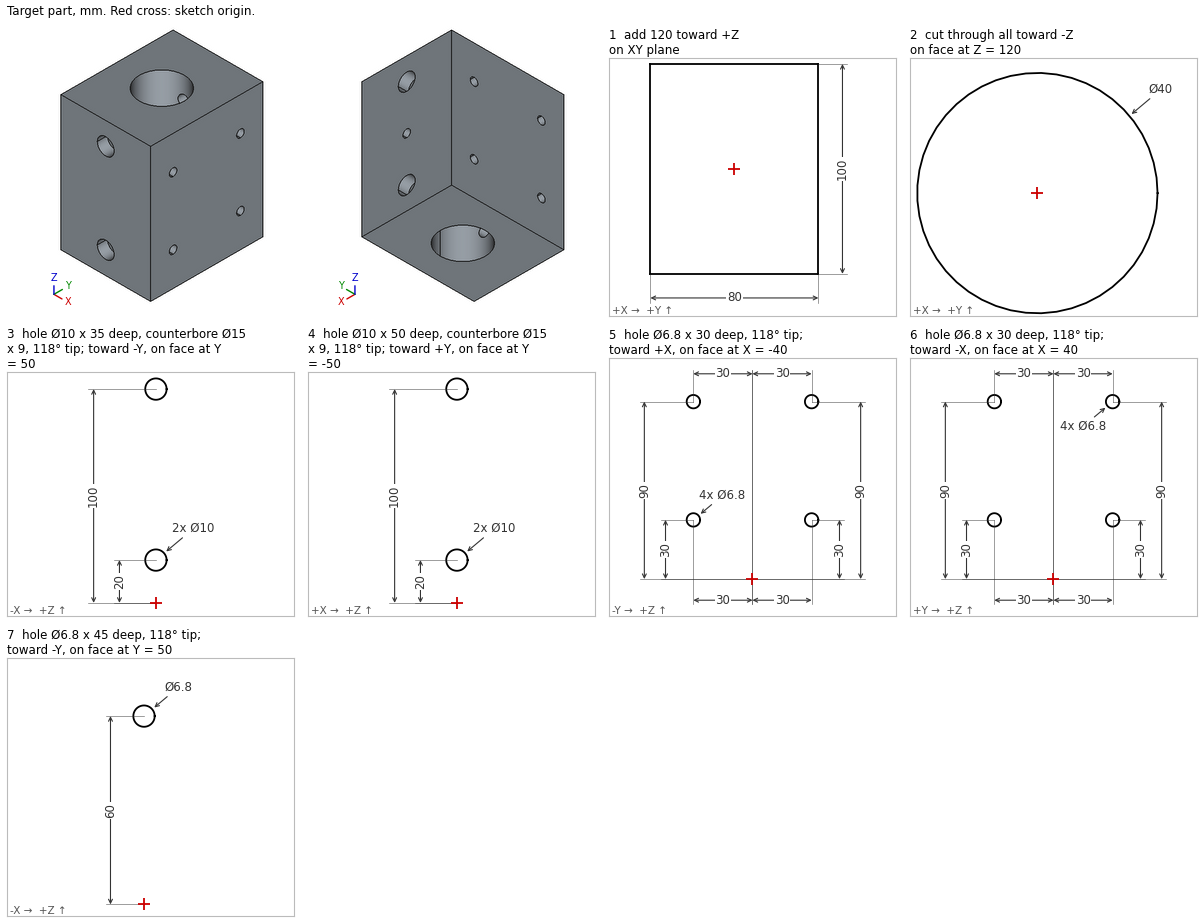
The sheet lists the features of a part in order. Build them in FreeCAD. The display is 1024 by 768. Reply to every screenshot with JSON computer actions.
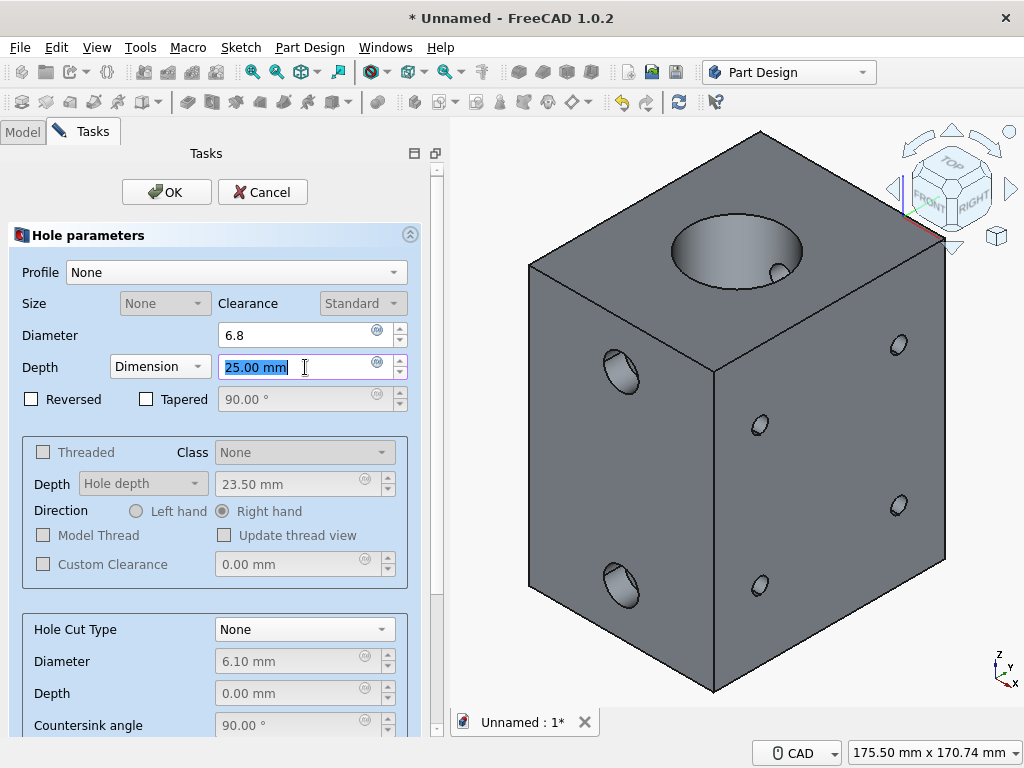
{"action": "type", "text": "30"}
{"action": "key", "text": "Tab"}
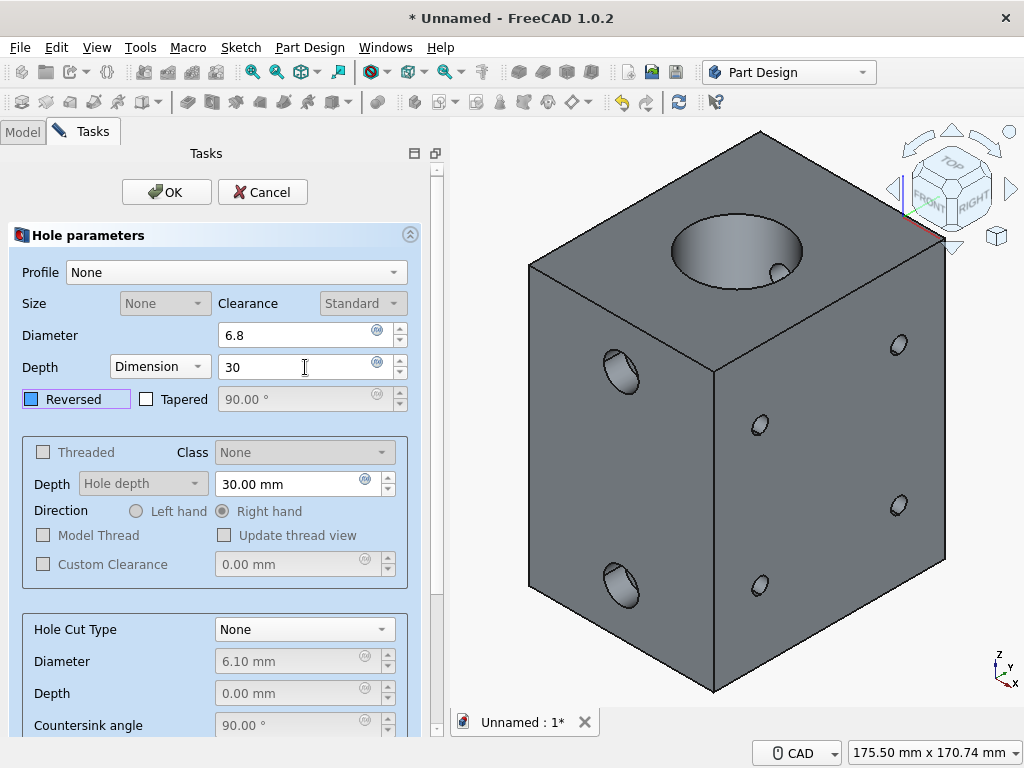
{"action": "left_click", "coordinate": [167, 192]}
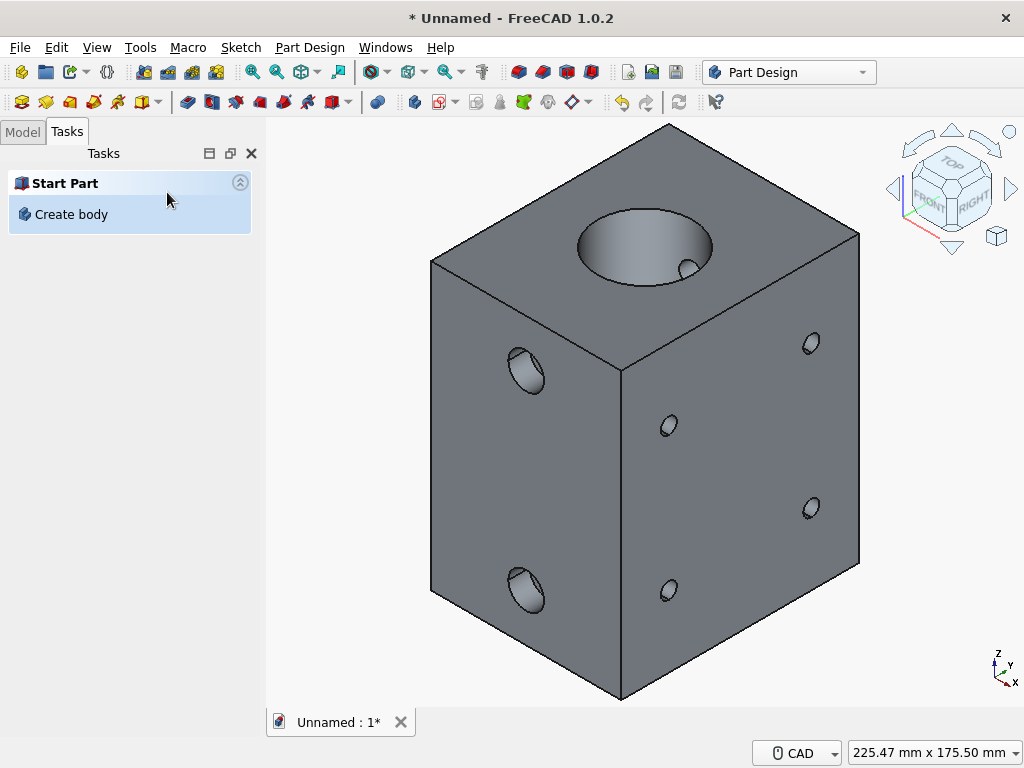
{"action": "key", "text": "4"}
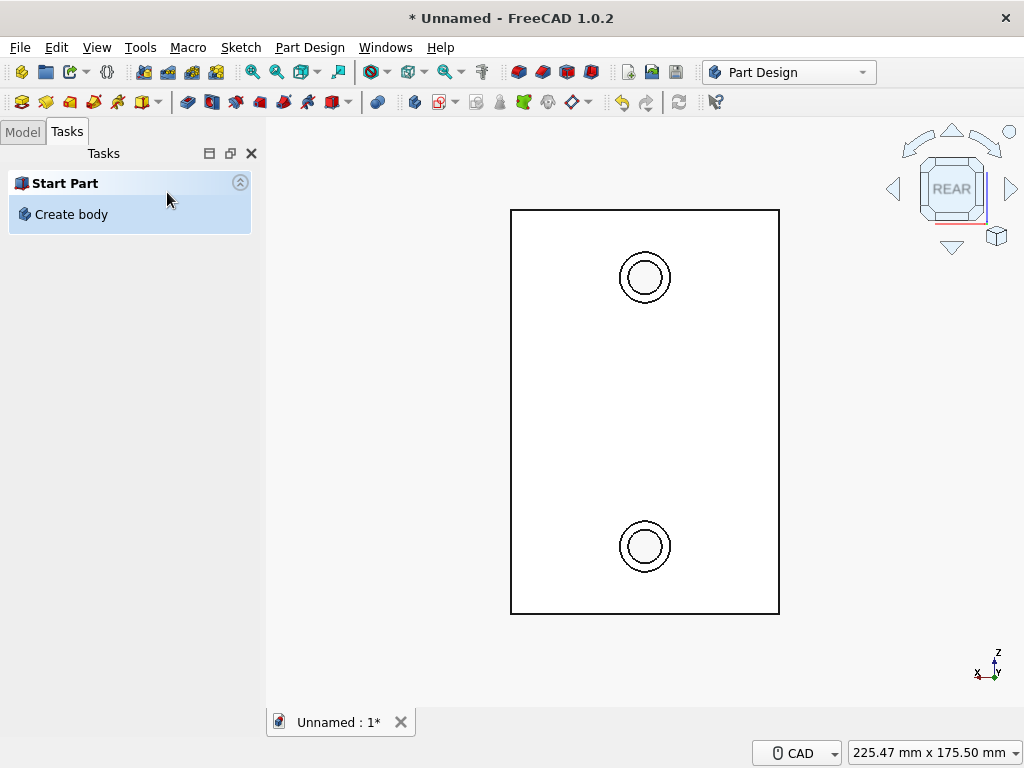
{"action": "left_click", "coordinate": [645, 411]}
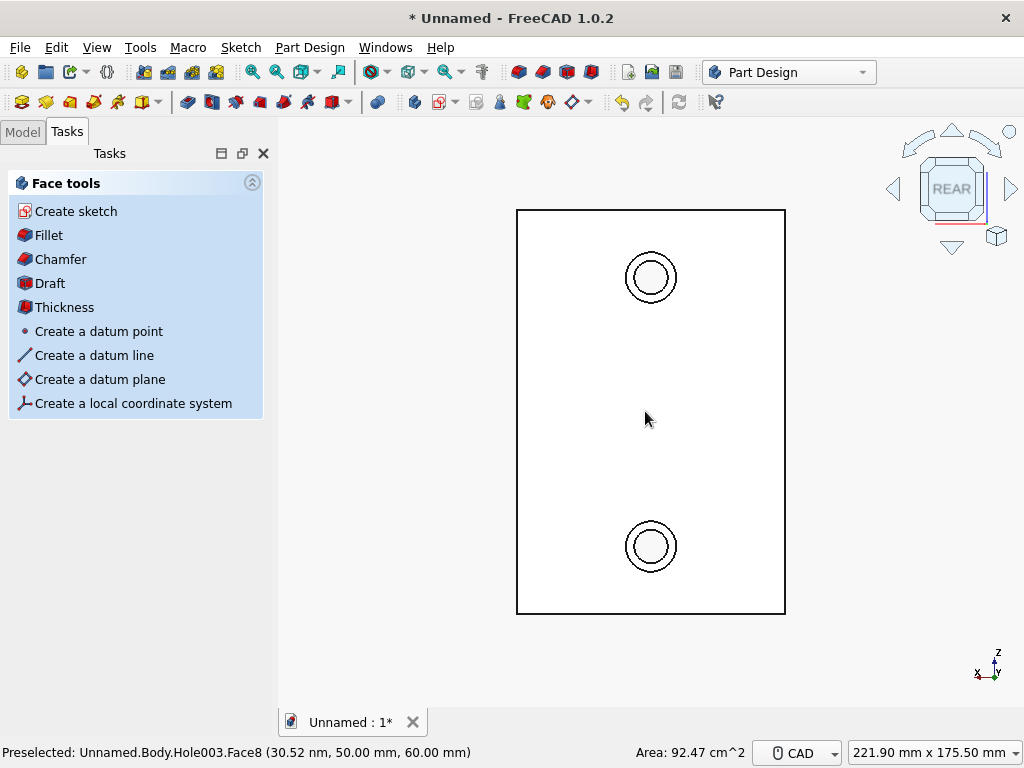
{"action": "left_click", "coordinate": [440, 102]}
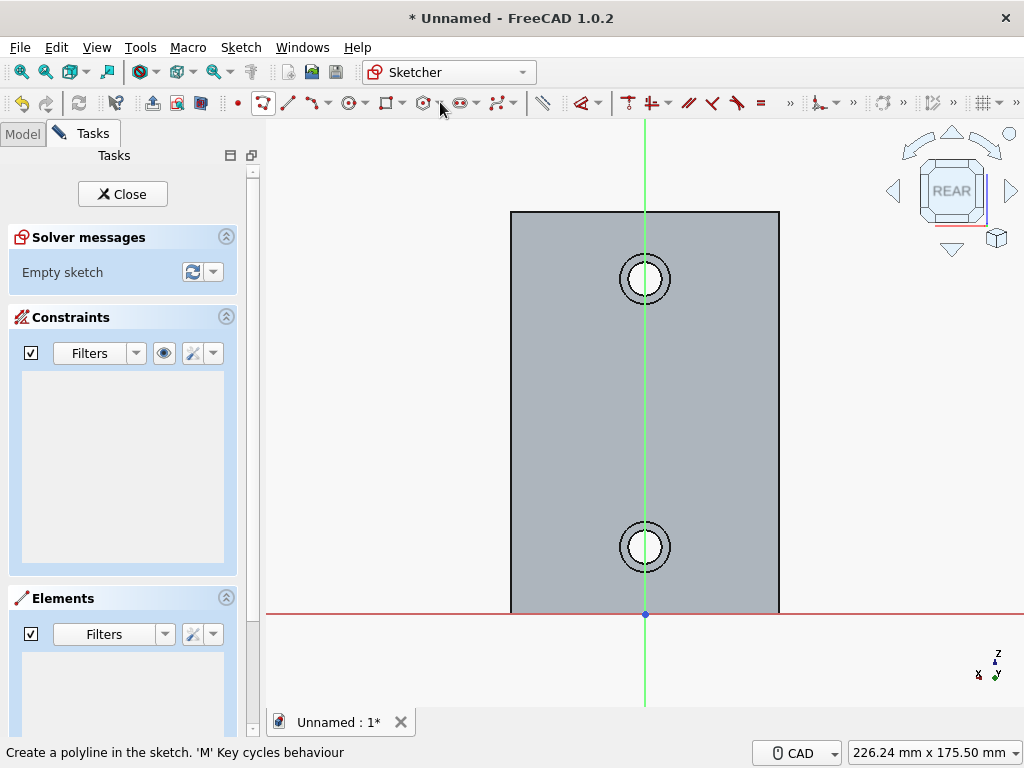
{"action": "scroll", "coordinate": [649, 413], "scroll_direction": "up", "scroll_amount": 14}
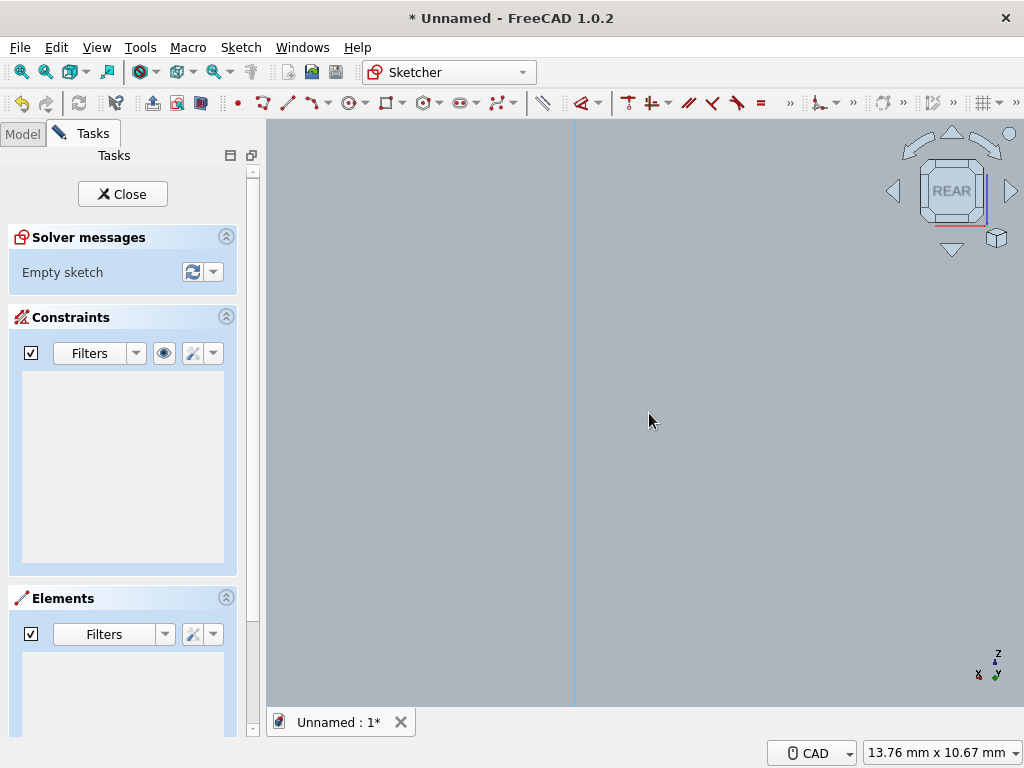
{"action": "left_click", "coordinate": [350, 104]}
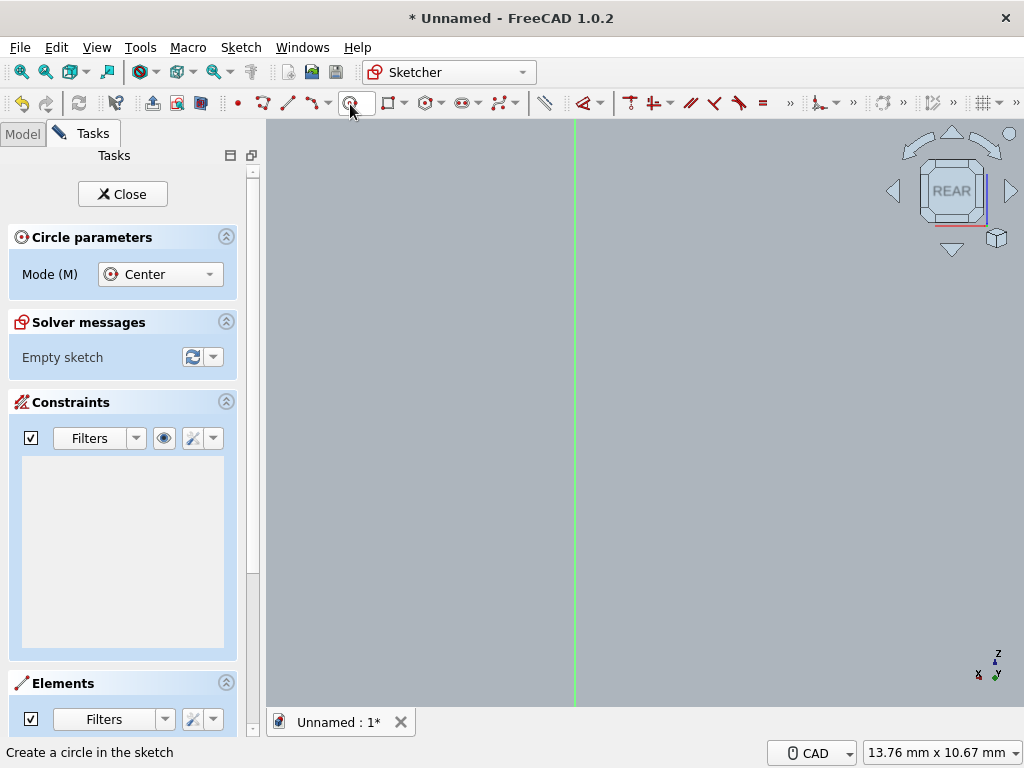
{"action": "left_click", "coordinate": [575, 405]}
{"action": "mouse_move", "coordinate": [708, 273]}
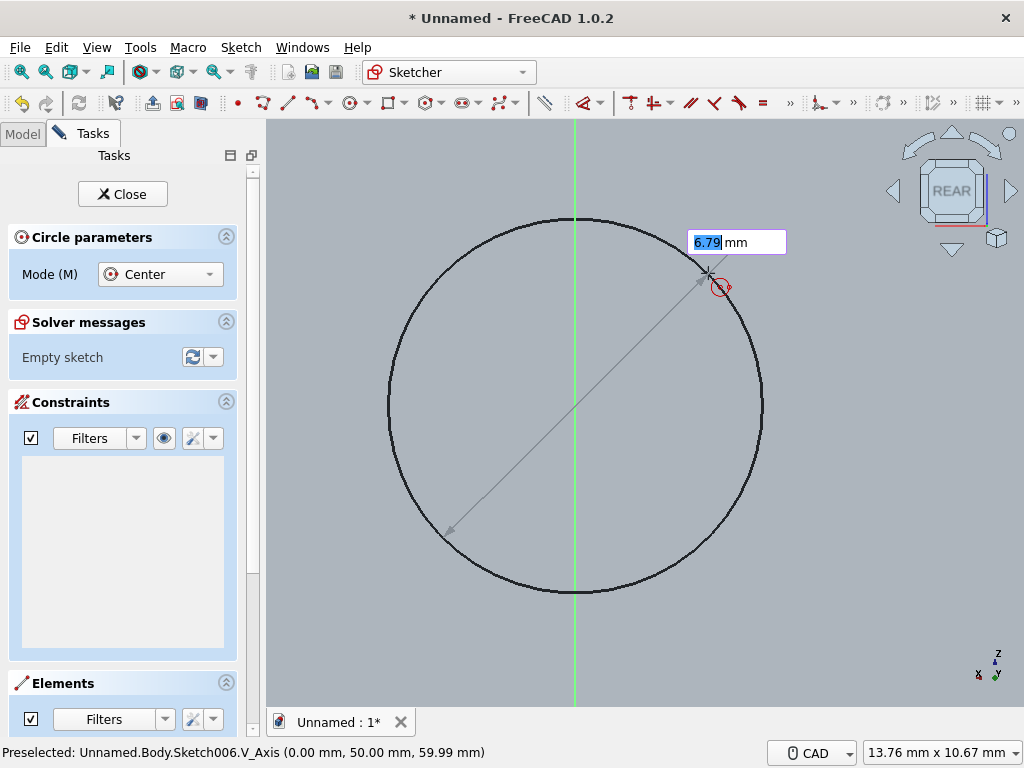
{"action": "type", "text": "6.8"}
{"action": "key", "text": "Return"}
{"action": "key", "text": "Escape"}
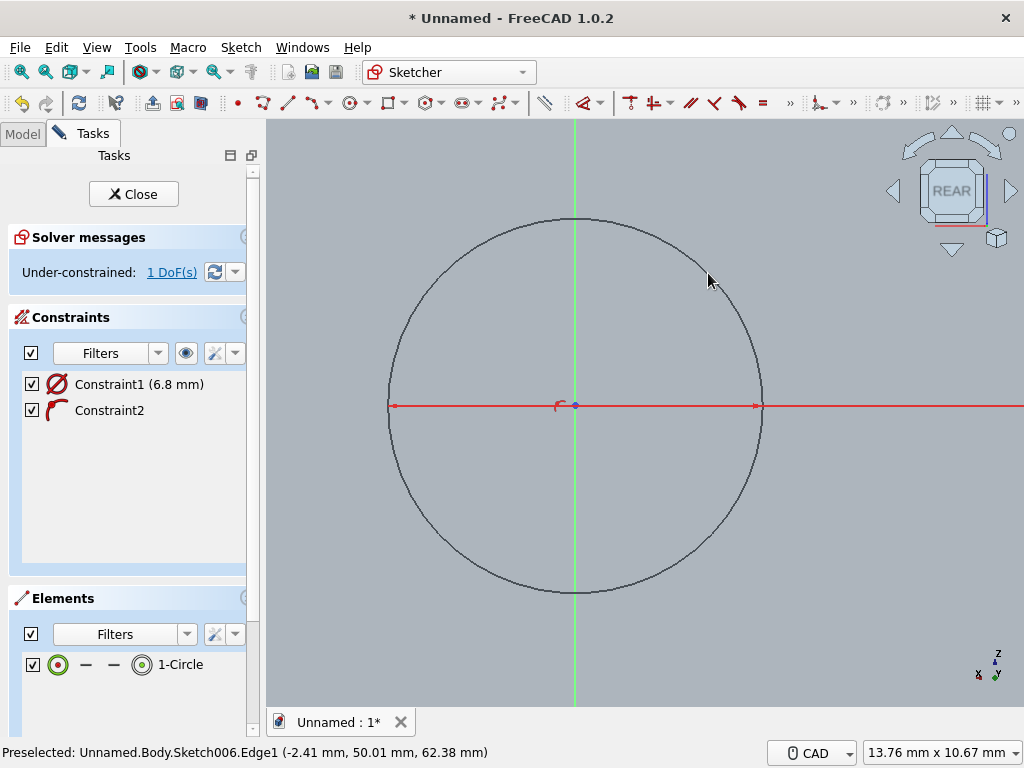
{"action": "left_click", "coordinate": [584, 104]}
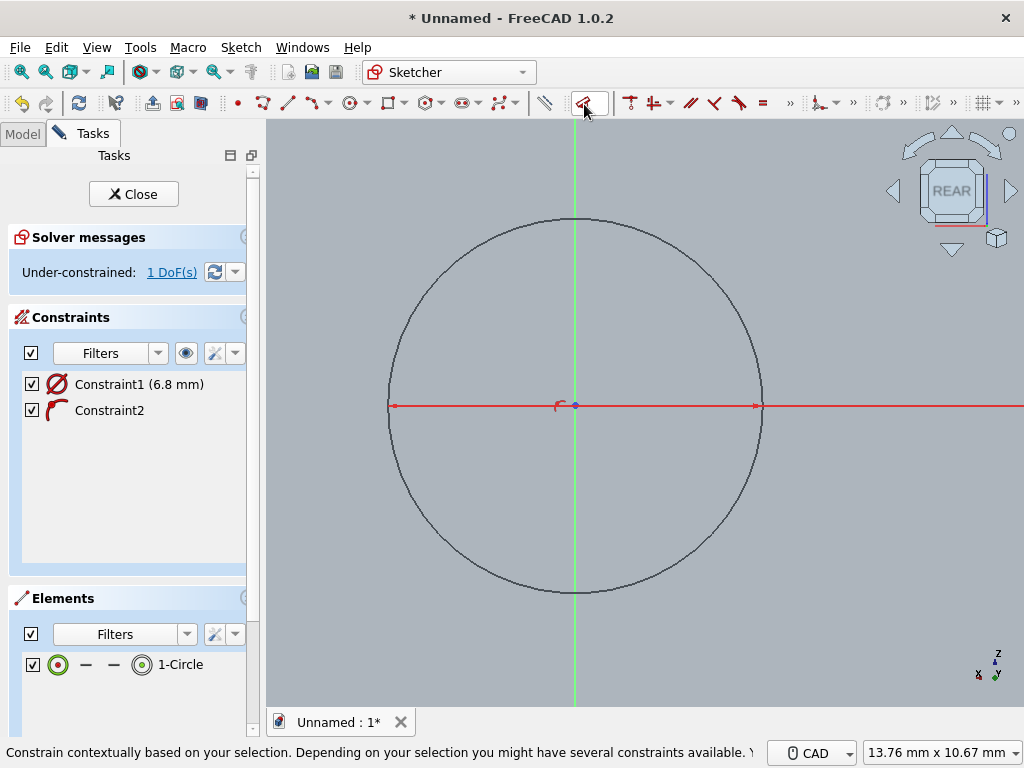
{"action": "left_click", "coordinate": [575, 406]}
{"action": "left_click", "coordinate": [609, 543]}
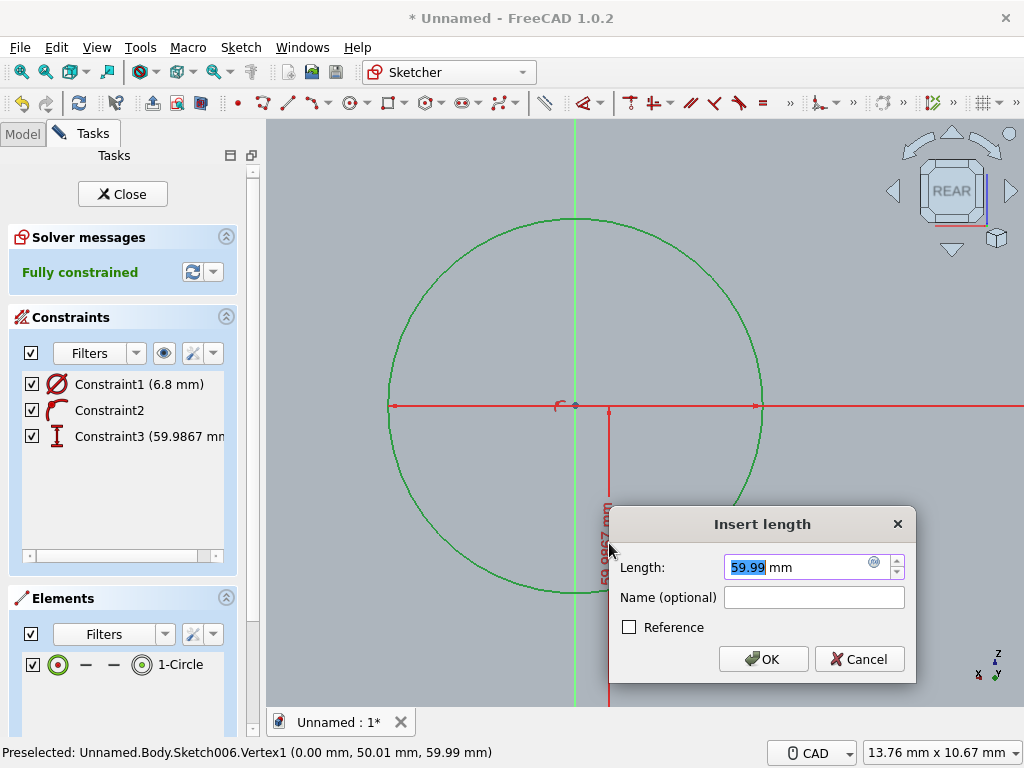
{"action": "type", "text": "60"}
{"action": "key", "text": "Return"}
{"action": "key", "text": "Escape"}